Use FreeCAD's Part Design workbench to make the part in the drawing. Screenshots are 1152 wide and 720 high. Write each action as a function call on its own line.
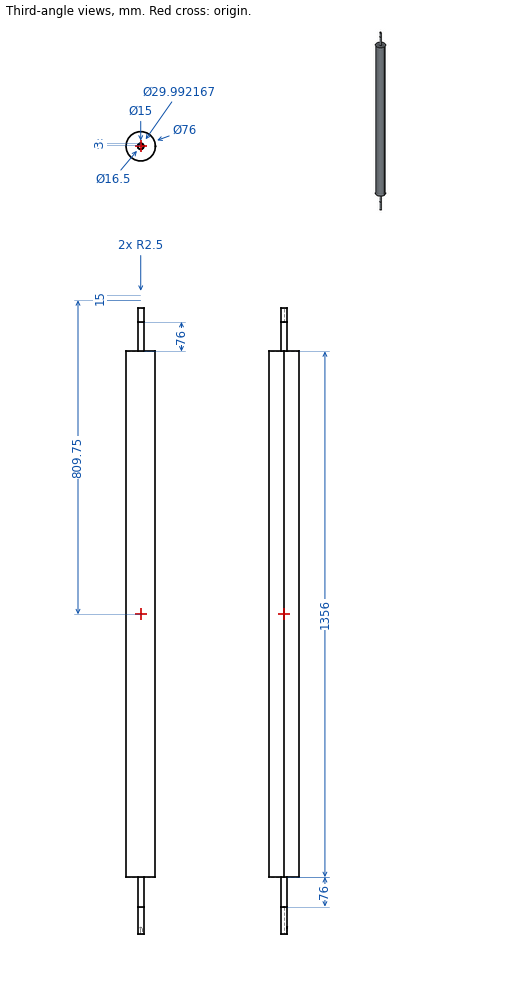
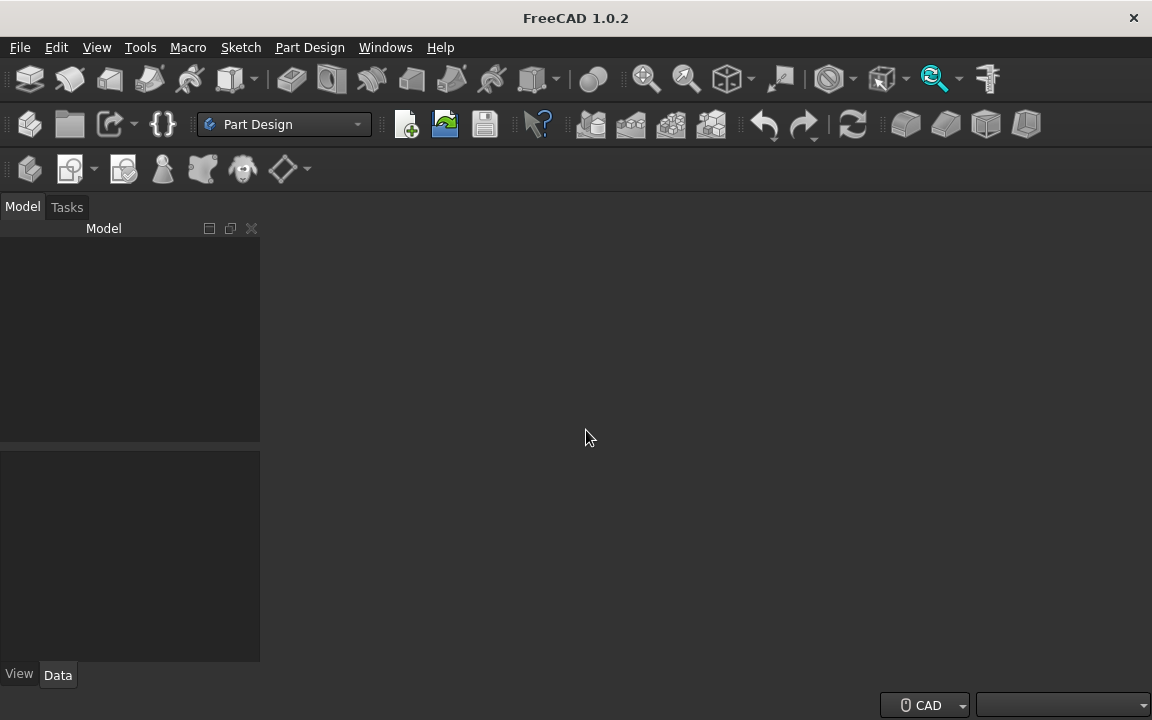
click(406, 124)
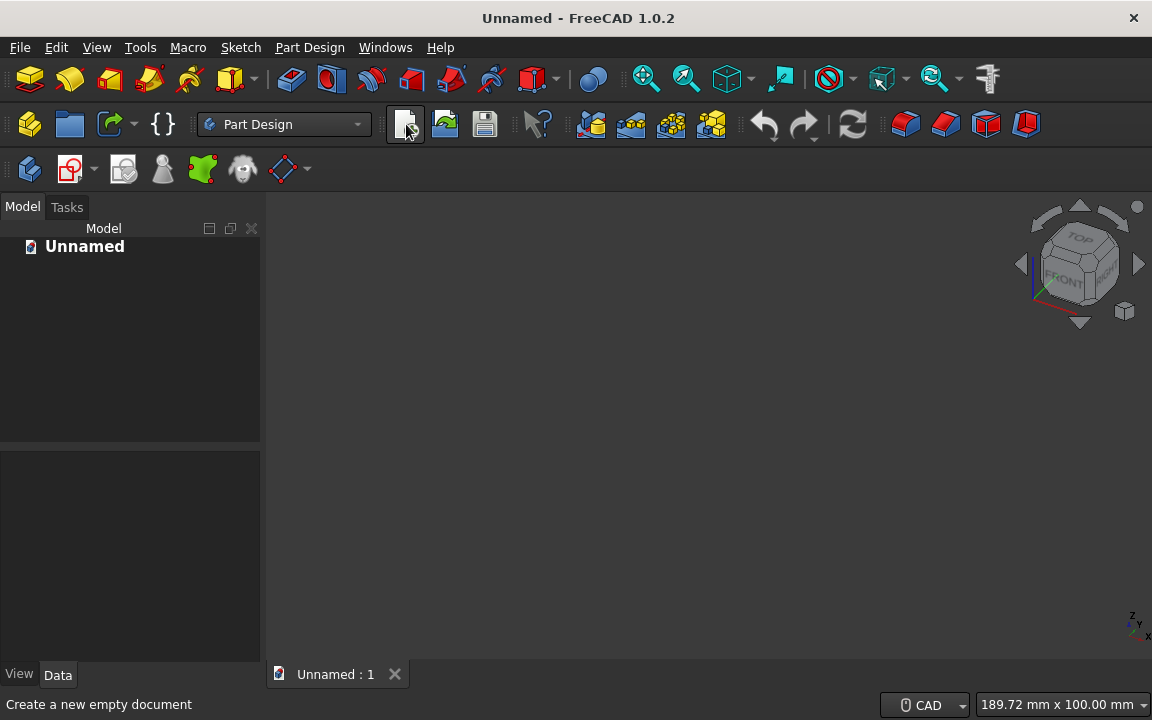
click(70, 170)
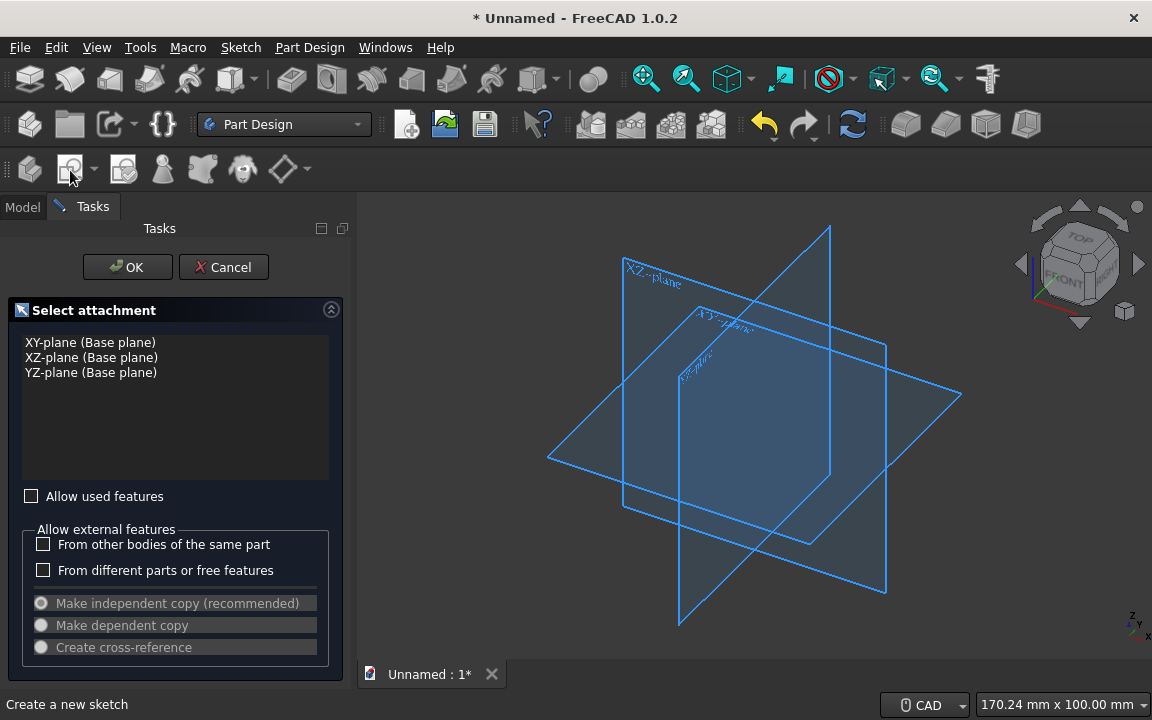
click(82, 342)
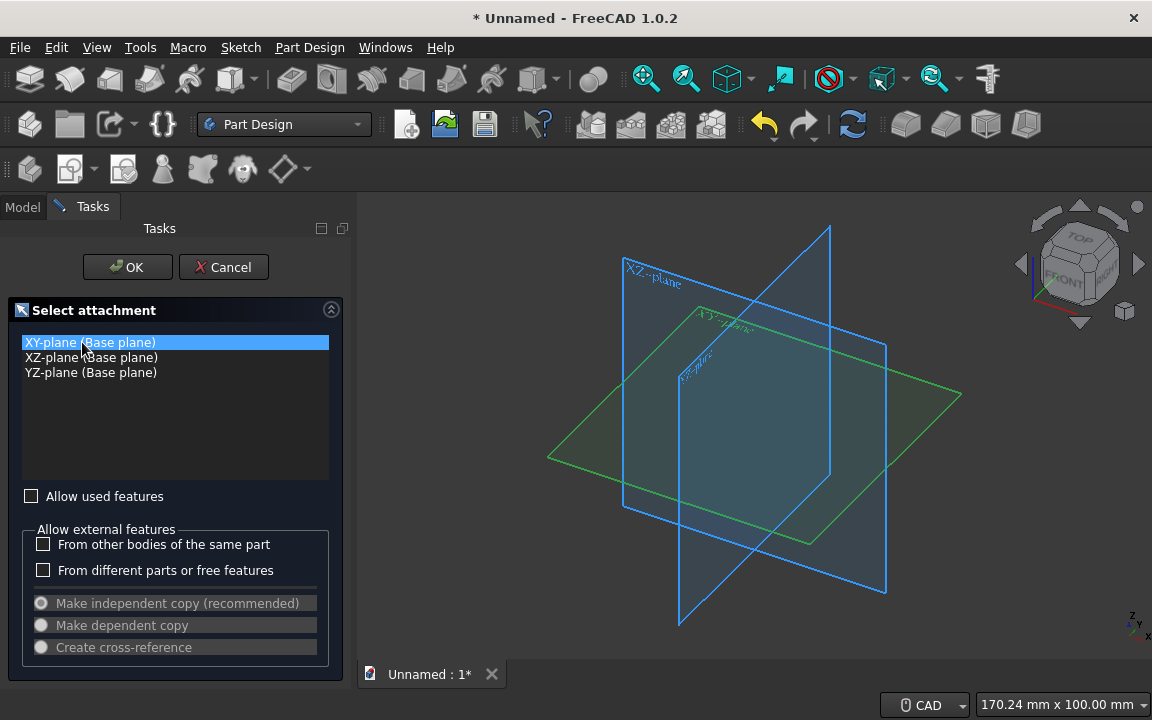
click(128, 267)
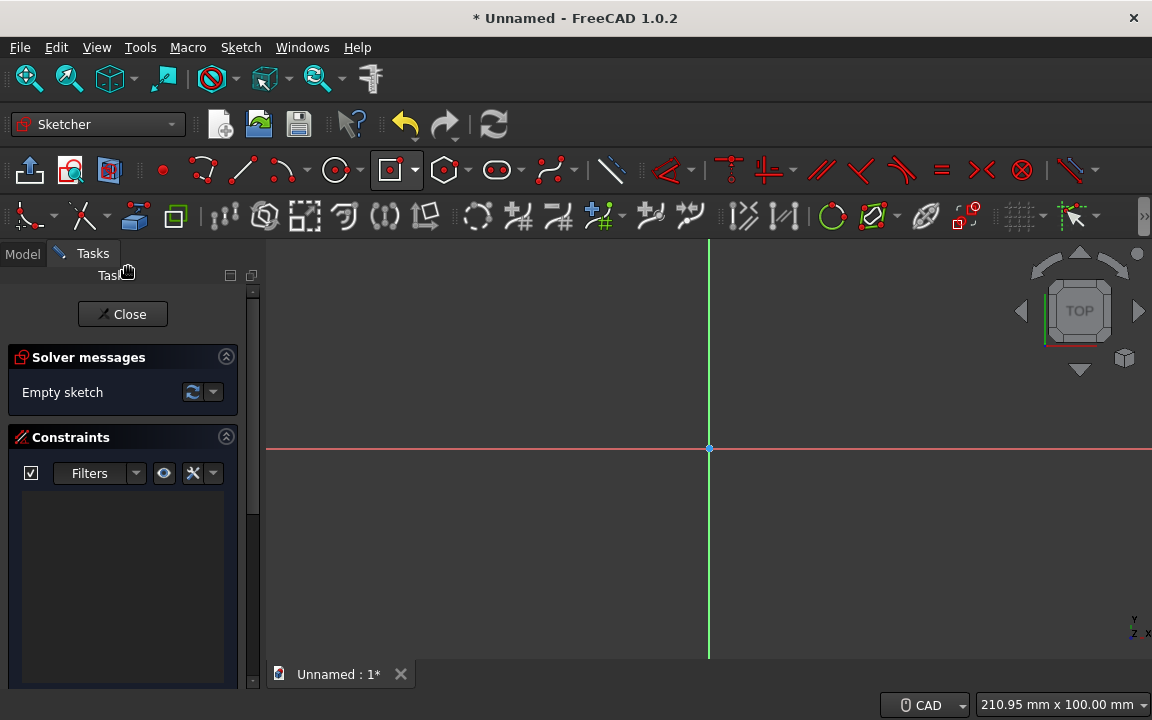
scroll(331, 449, down, 1)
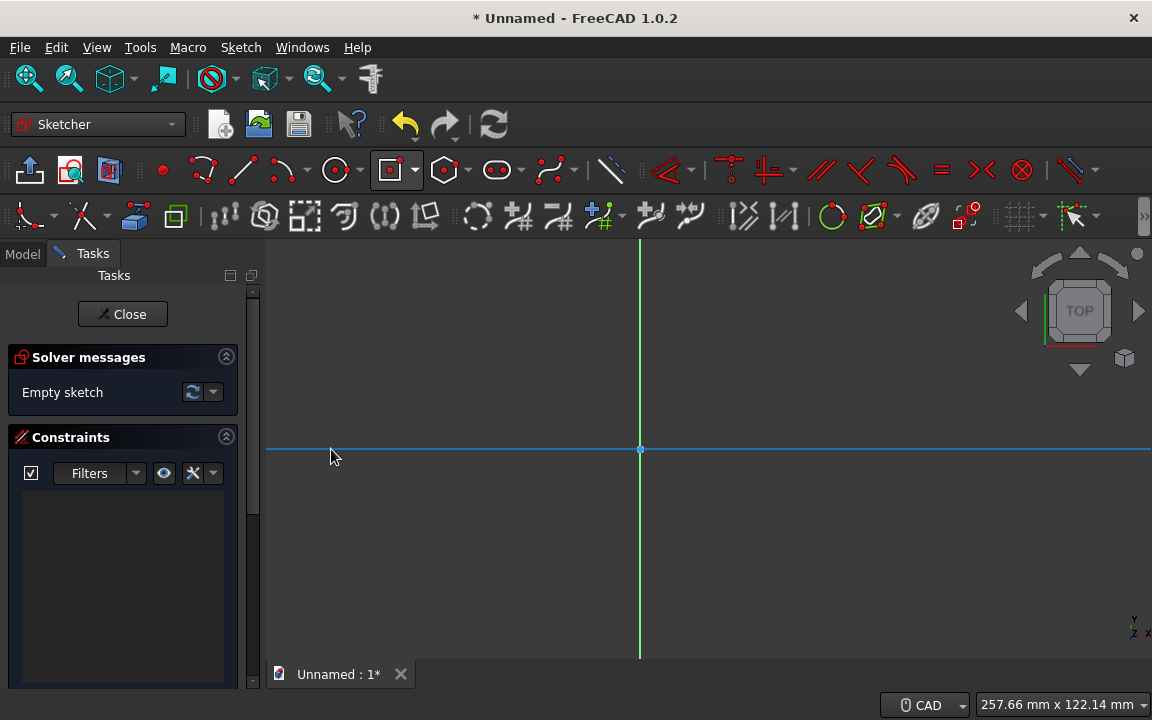
click(336, 170)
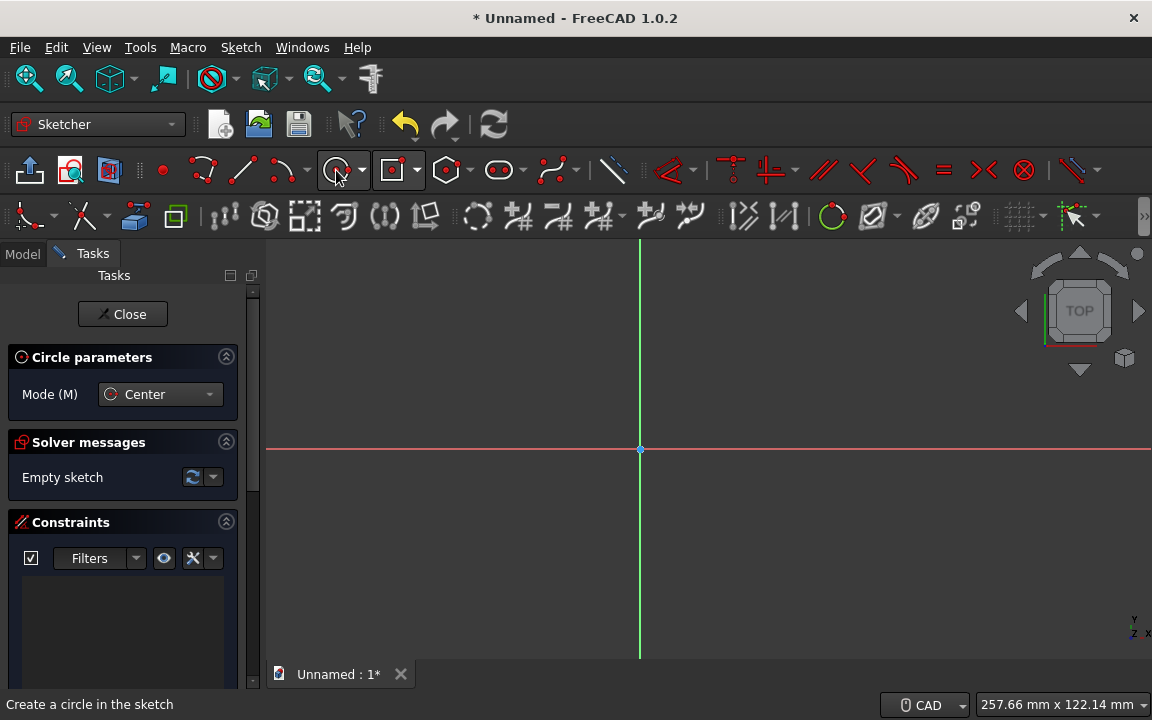
click(640, 449)
click(733, 357)
key(Escape)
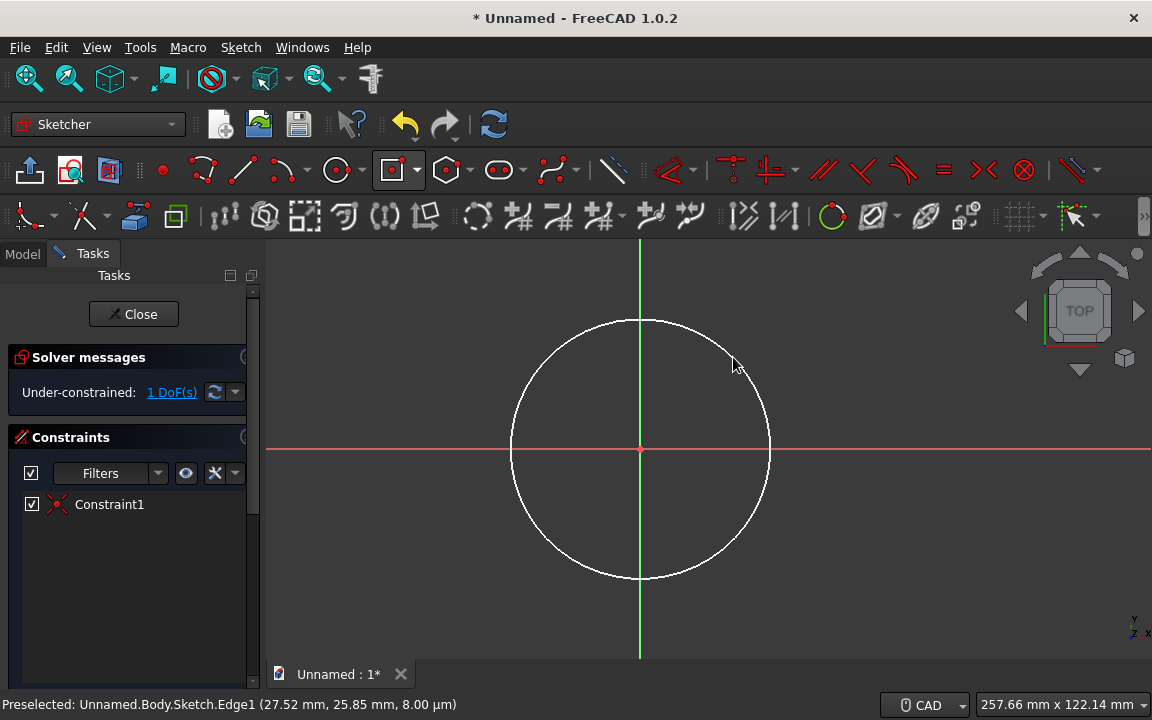
click(732, 357)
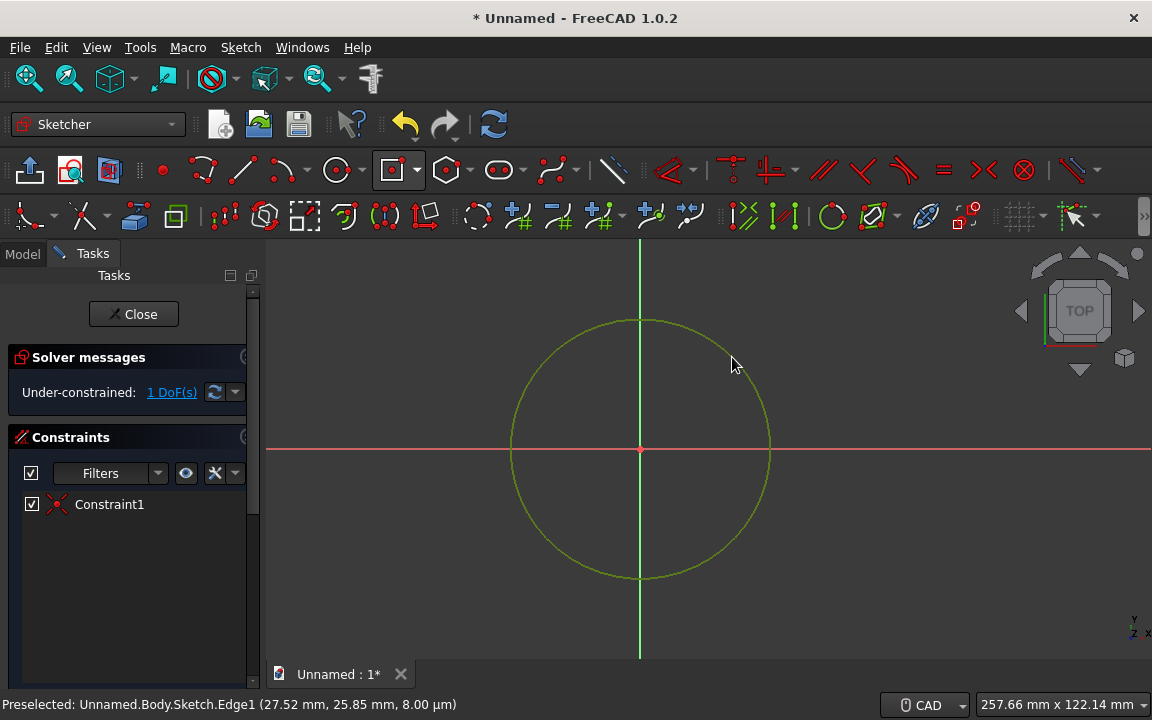
key(k)
key(o)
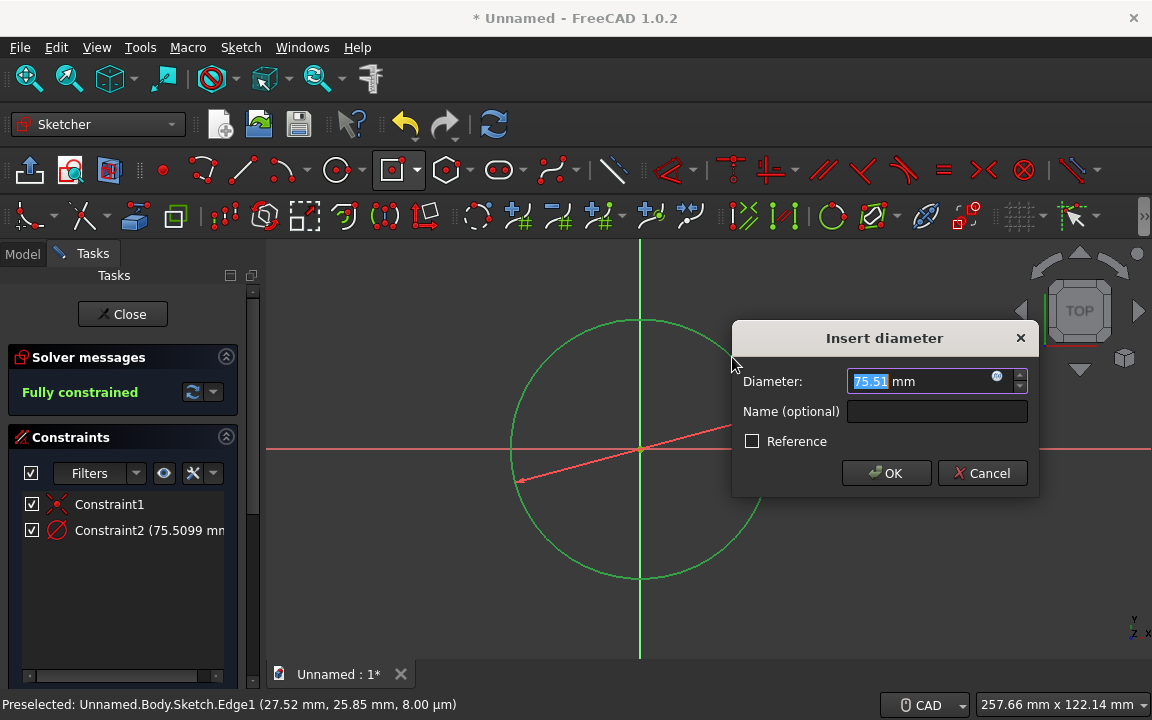
text(76)
key(Return)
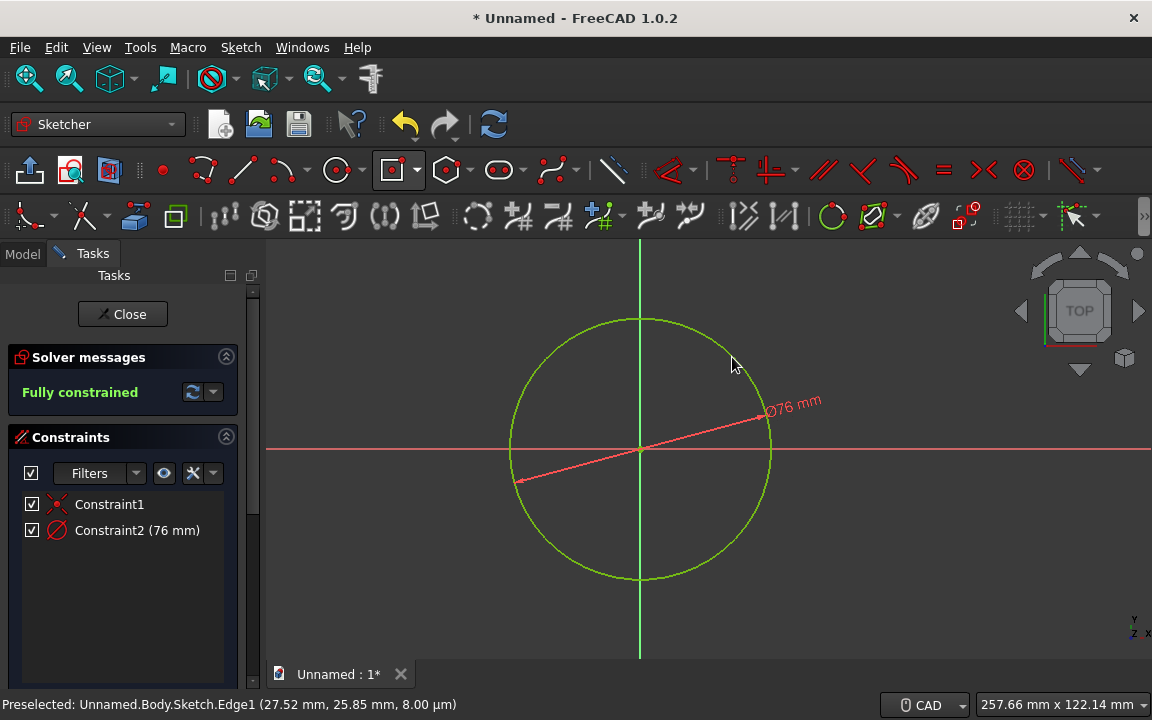
click(123, 314)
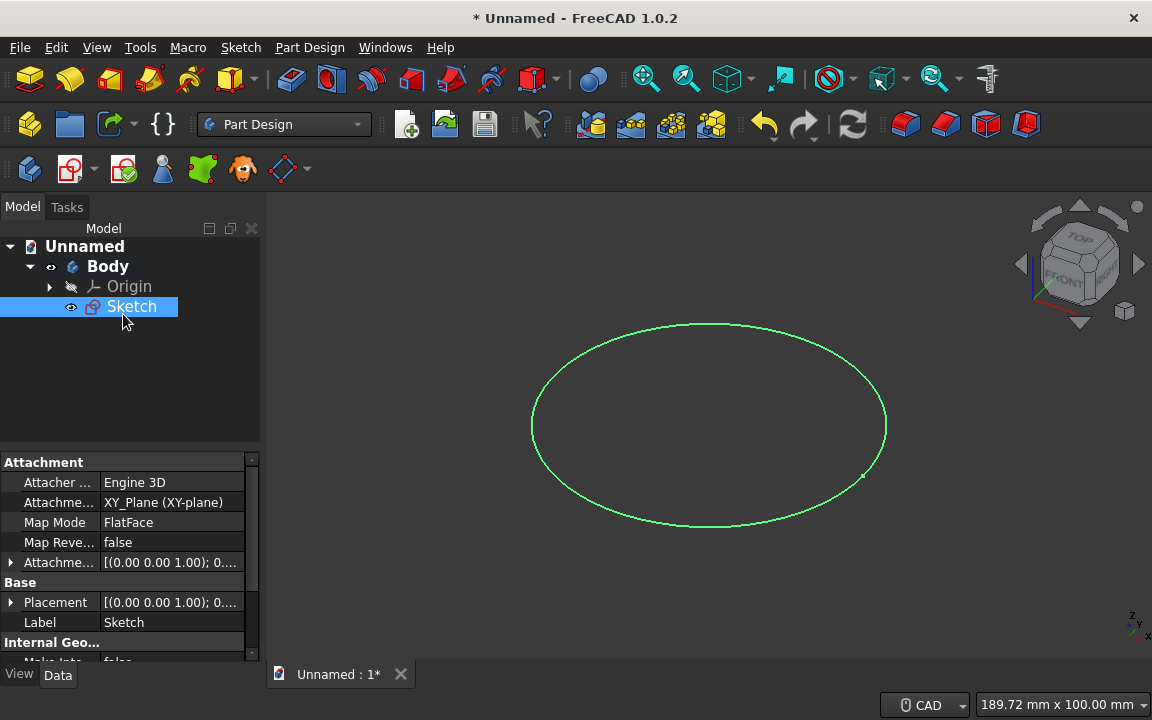
click(30, 80)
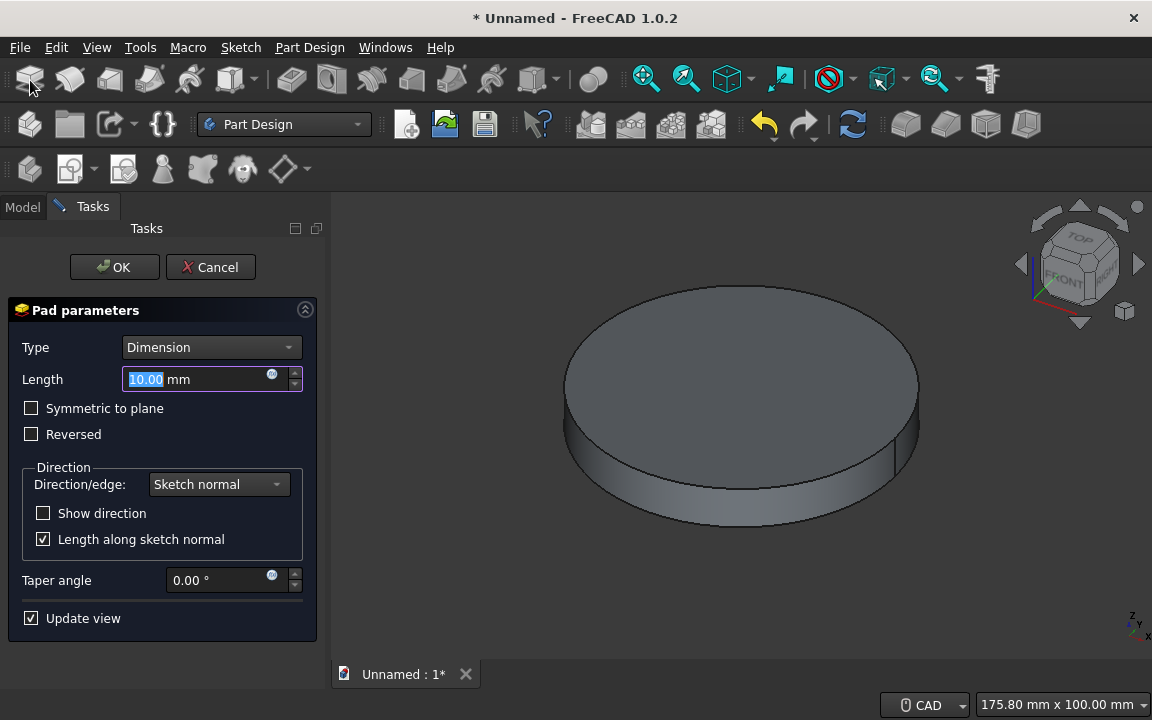
text(1356)
key(Tab)